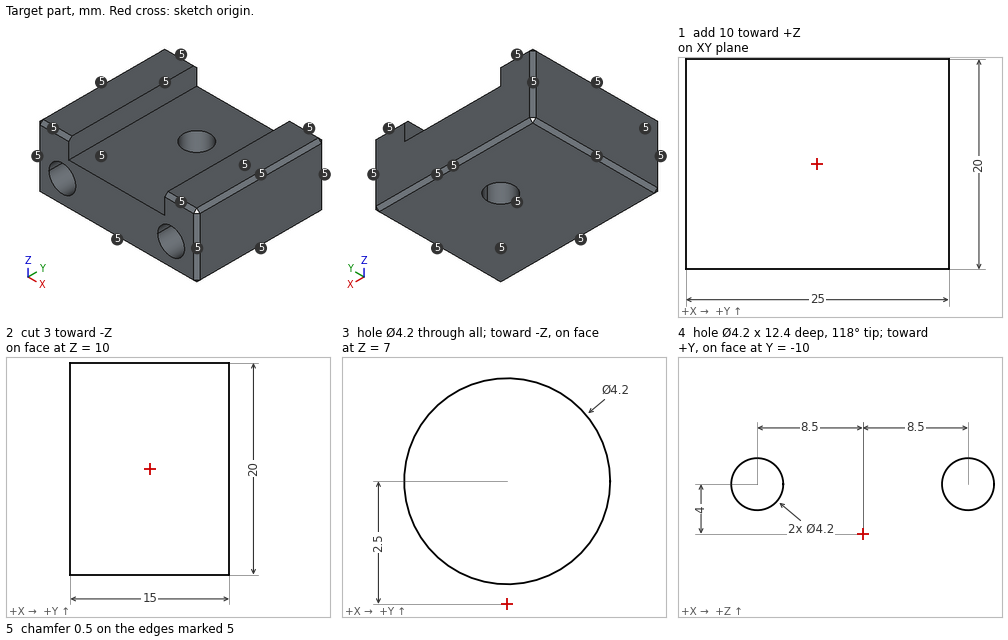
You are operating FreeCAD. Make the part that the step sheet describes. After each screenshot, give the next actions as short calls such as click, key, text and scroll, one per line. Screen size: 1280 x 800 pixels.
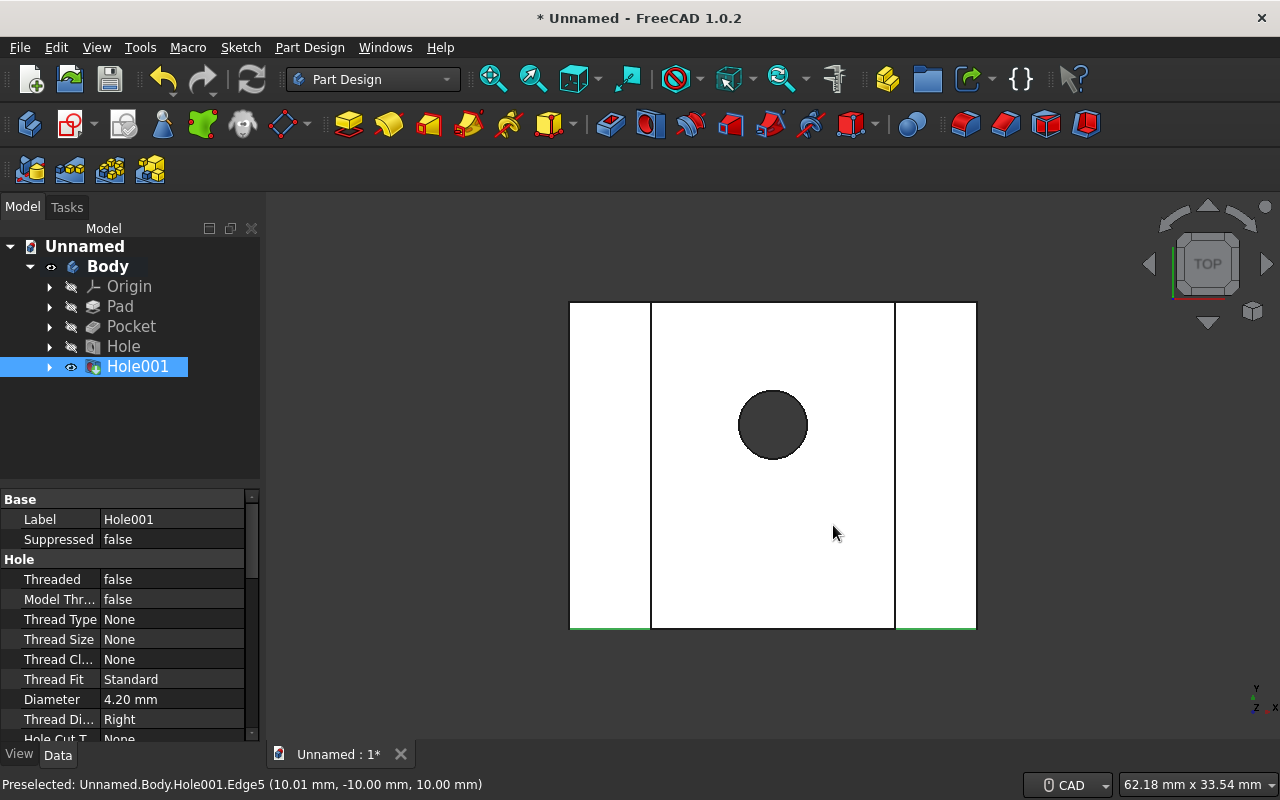
click(610, 301, ctrl)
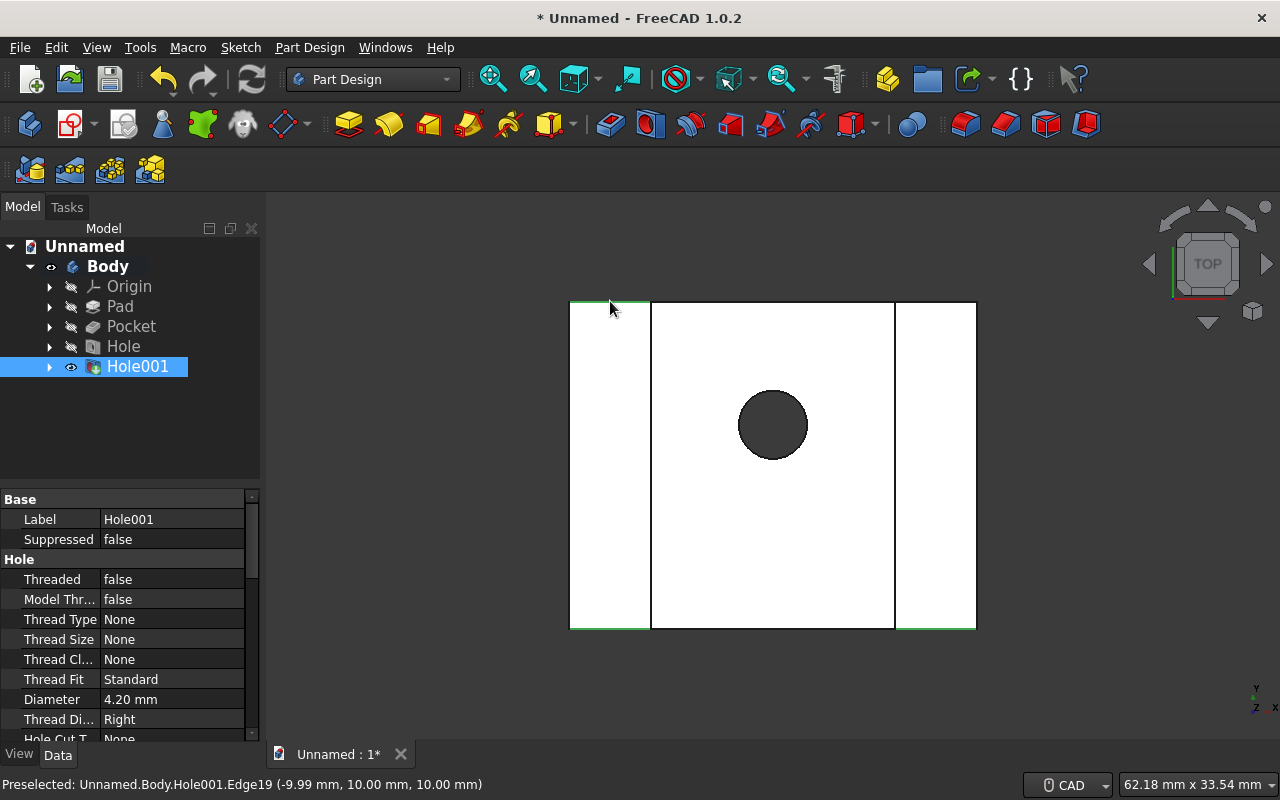
click(936, 301, ctrl)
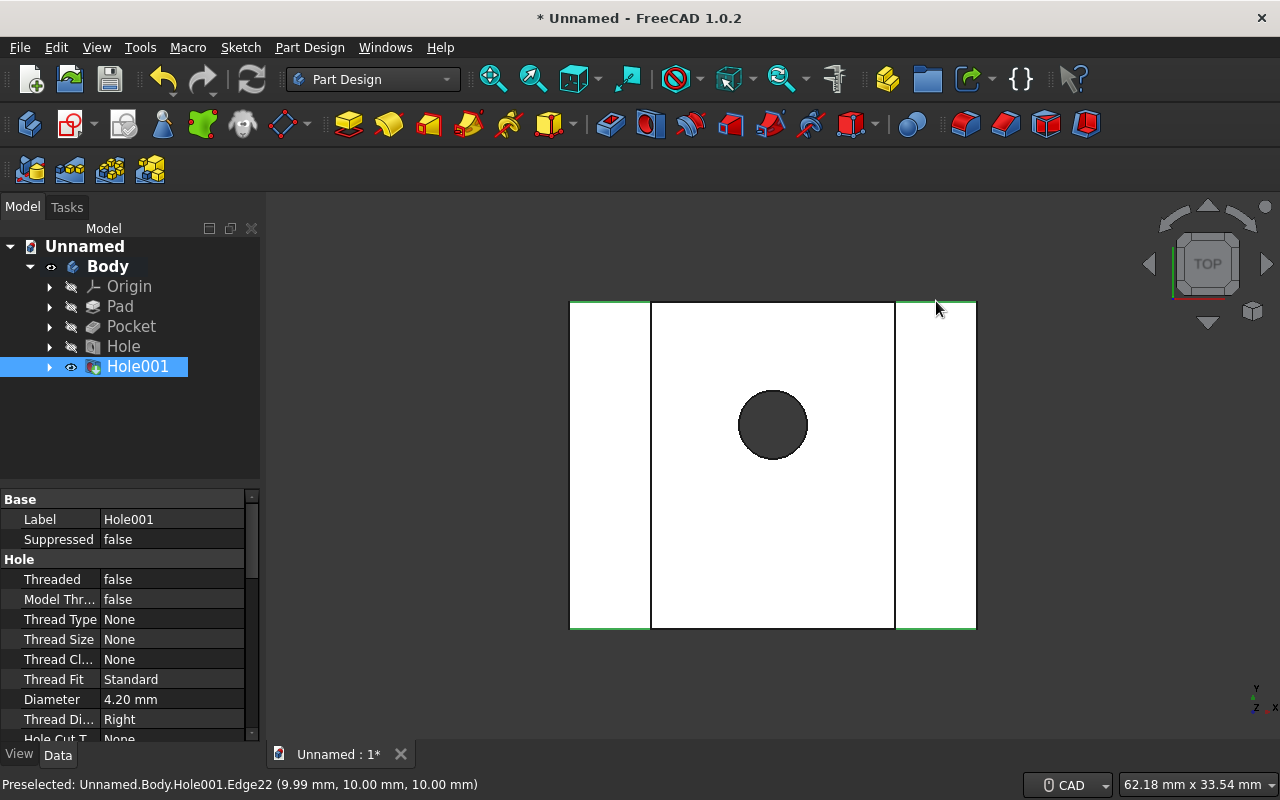
key(1)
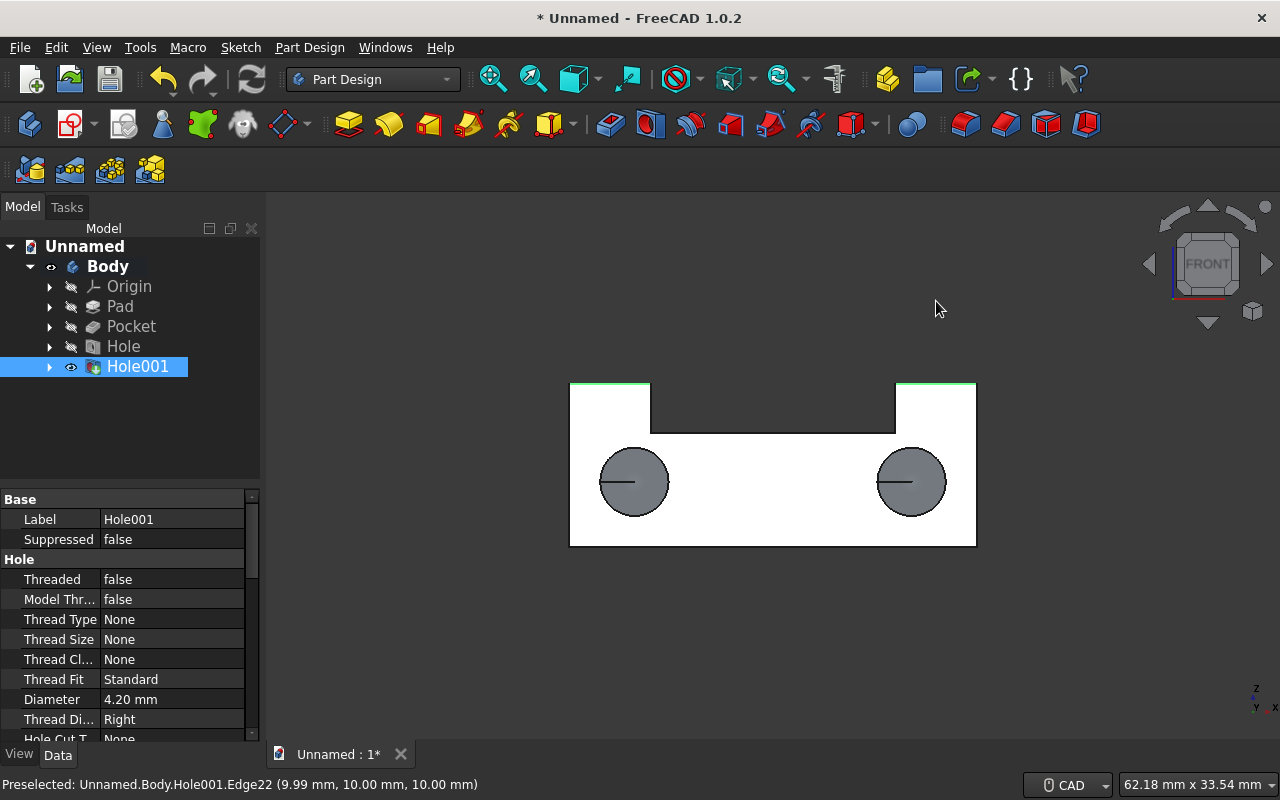
key(v)
key(f)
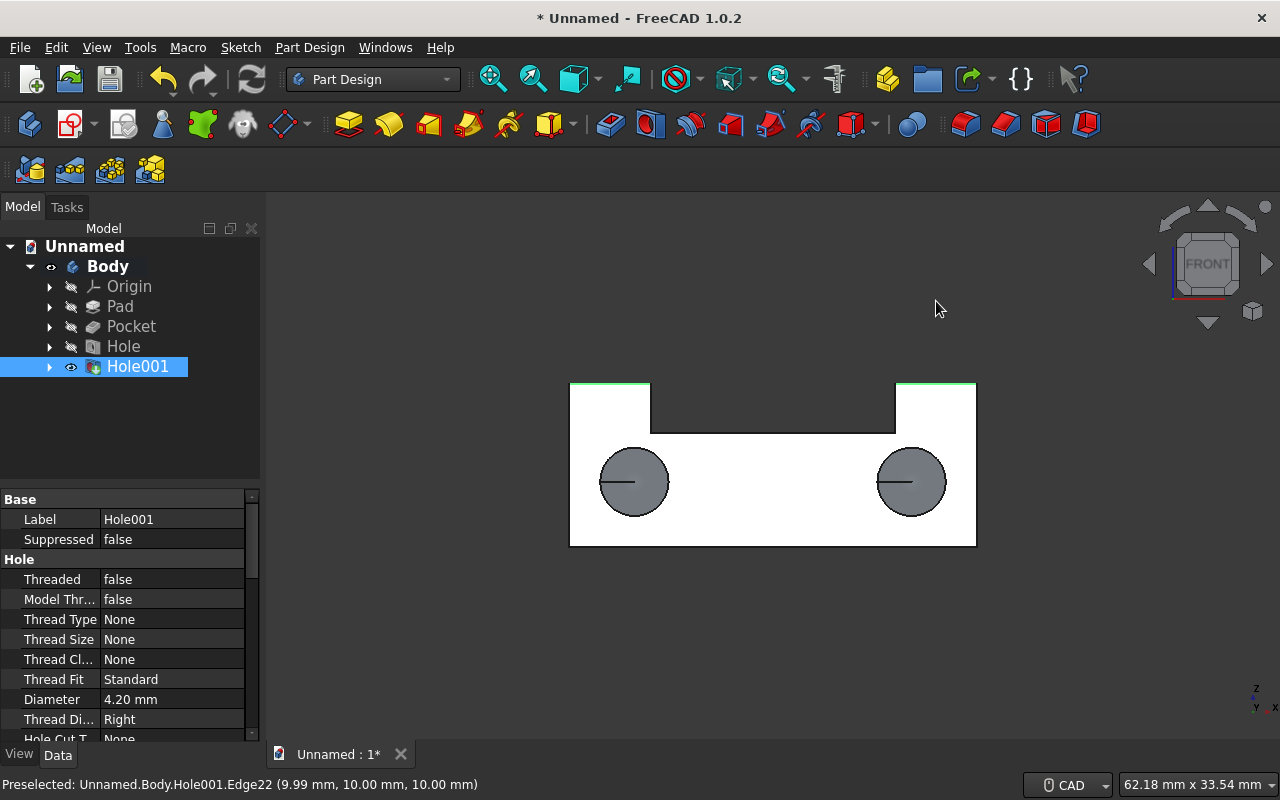
click(773, 546, ctrl)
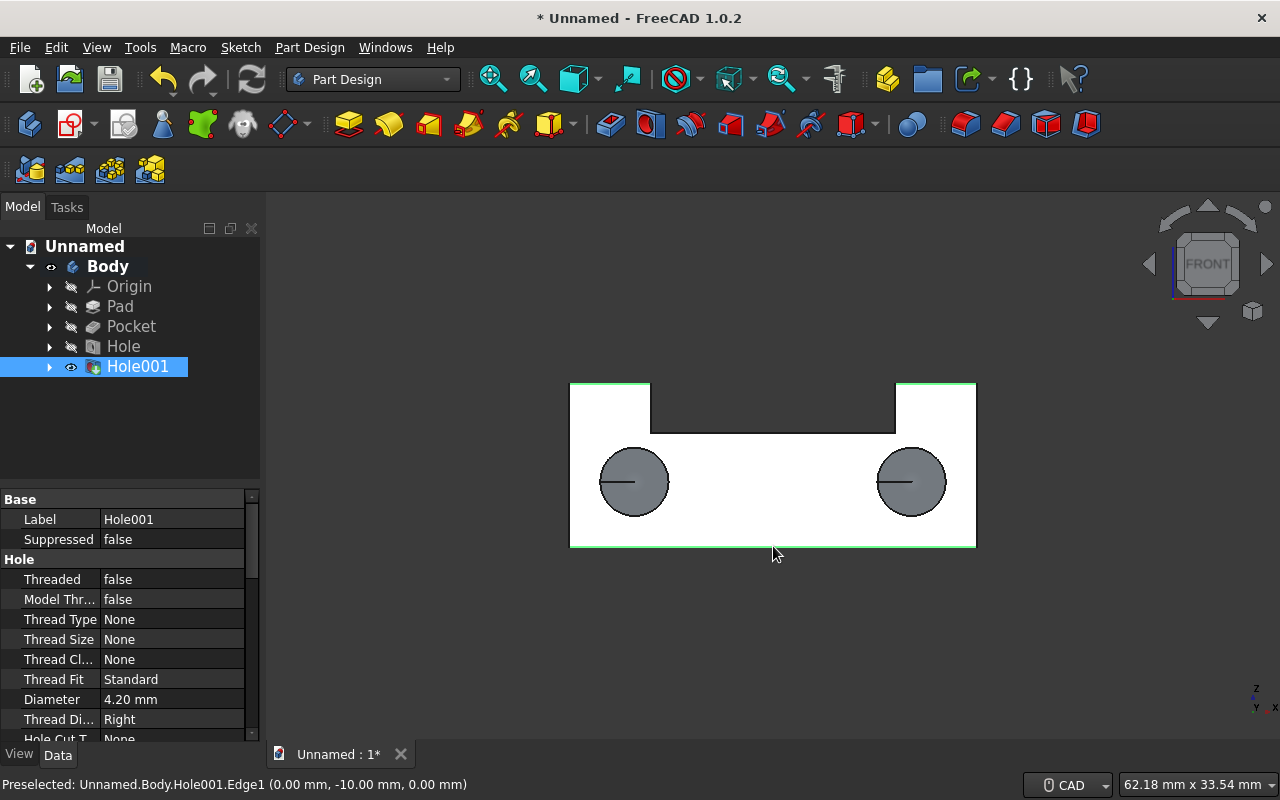
key(3)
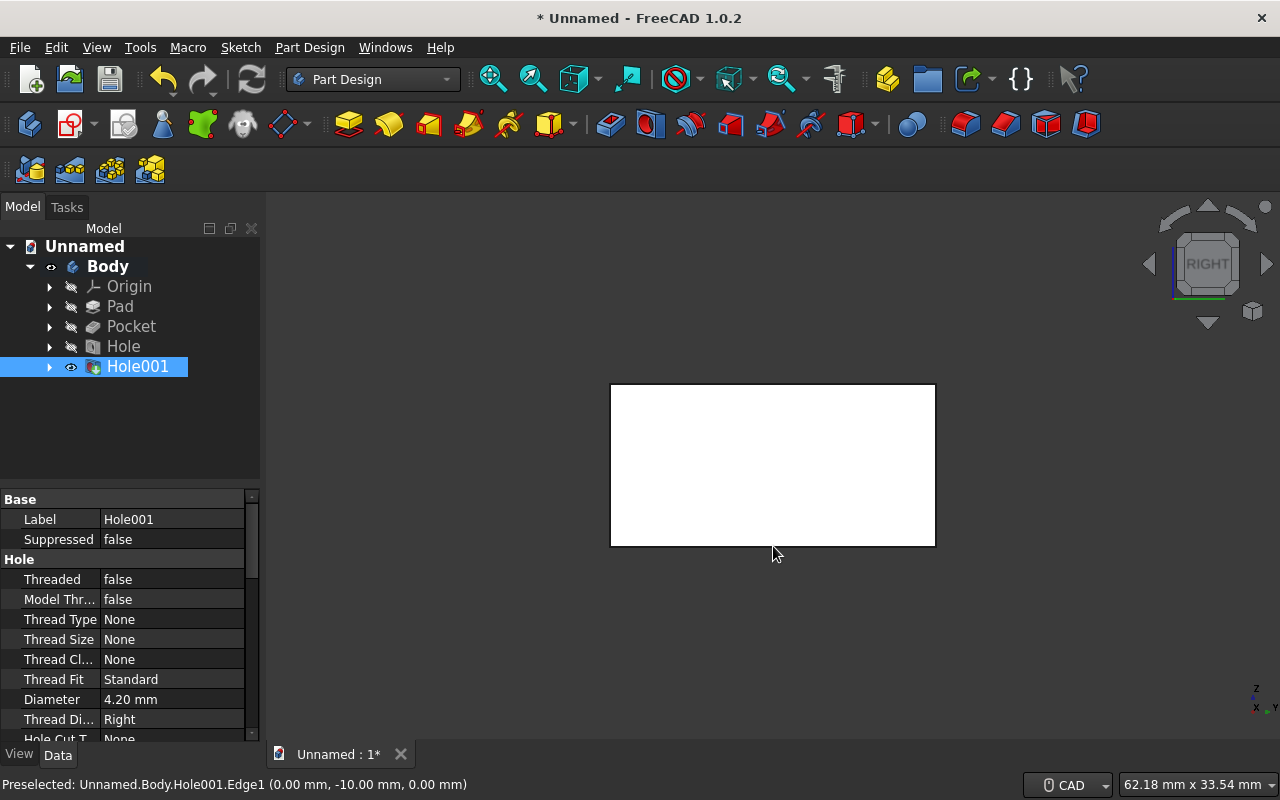
key(v)
key(f)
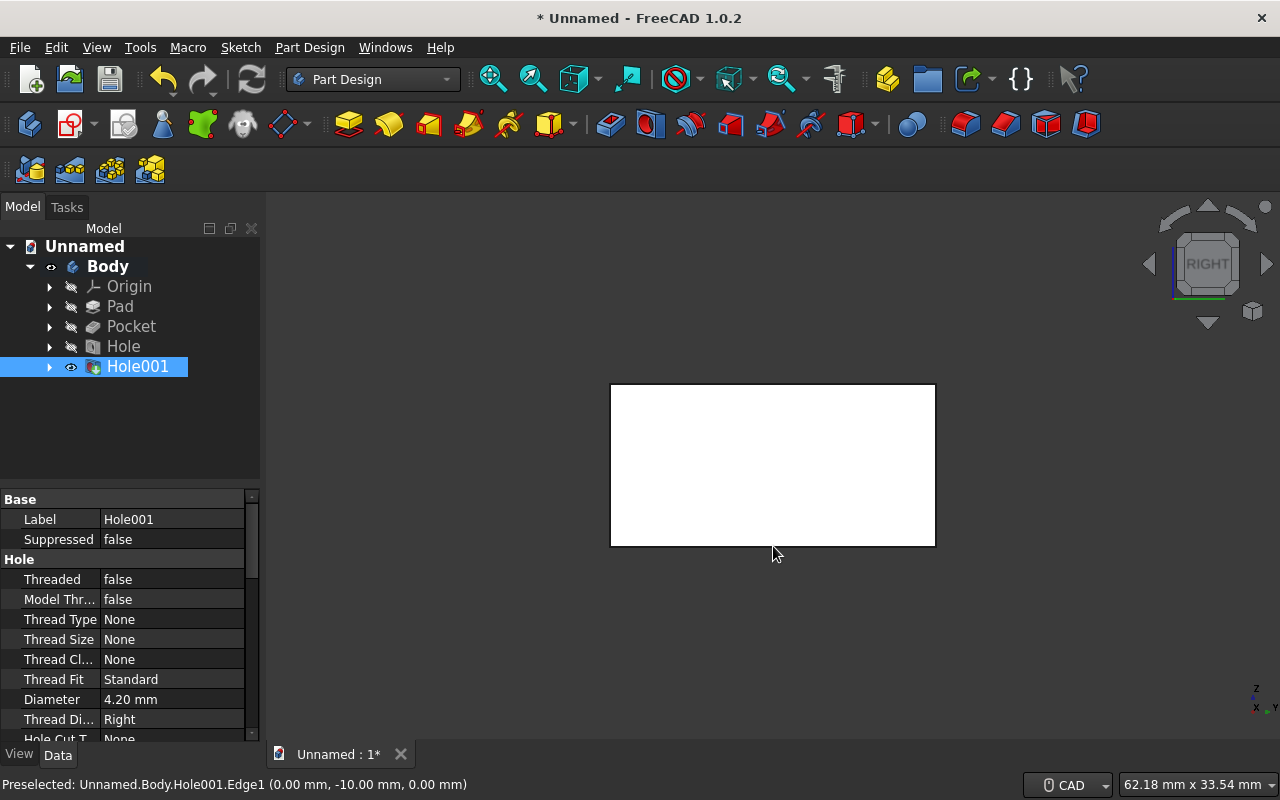
key(5)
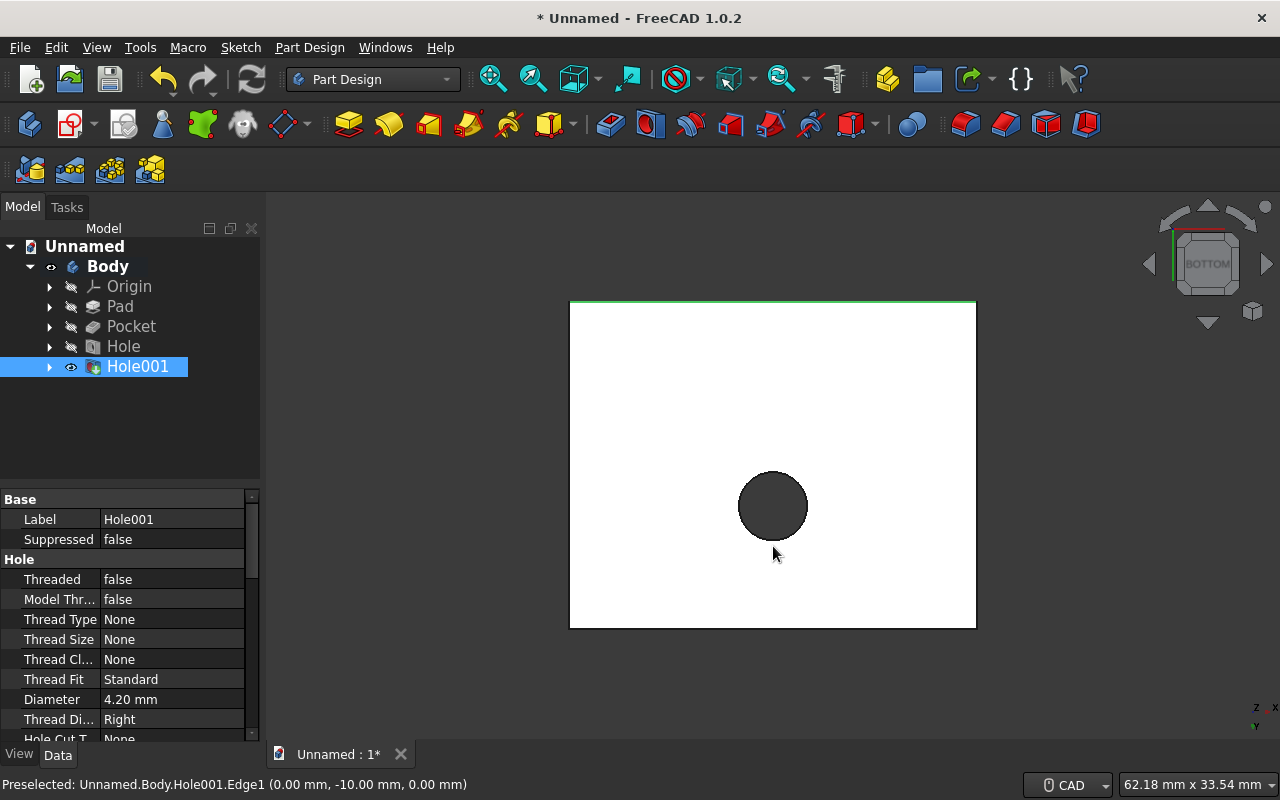
click(773, 628, ctrl)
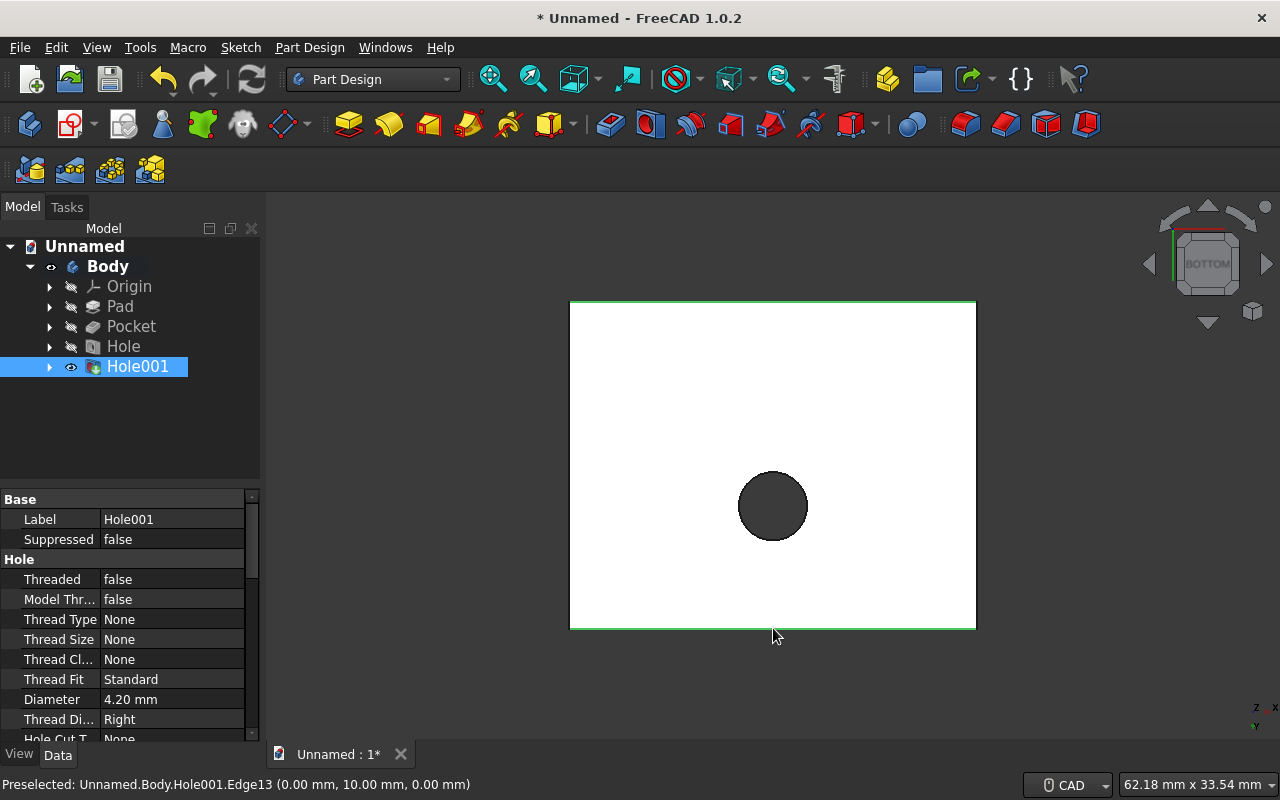
key(4)